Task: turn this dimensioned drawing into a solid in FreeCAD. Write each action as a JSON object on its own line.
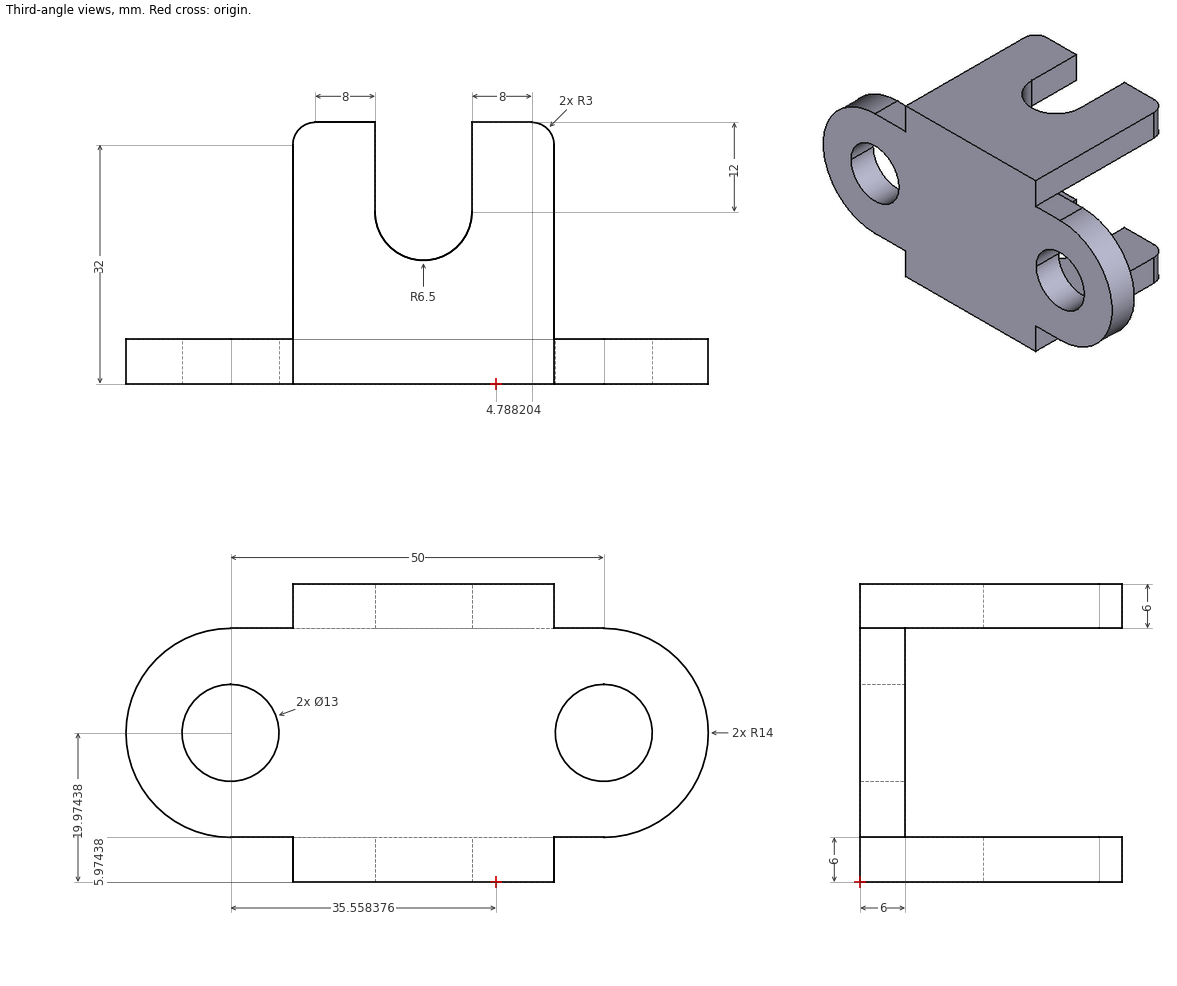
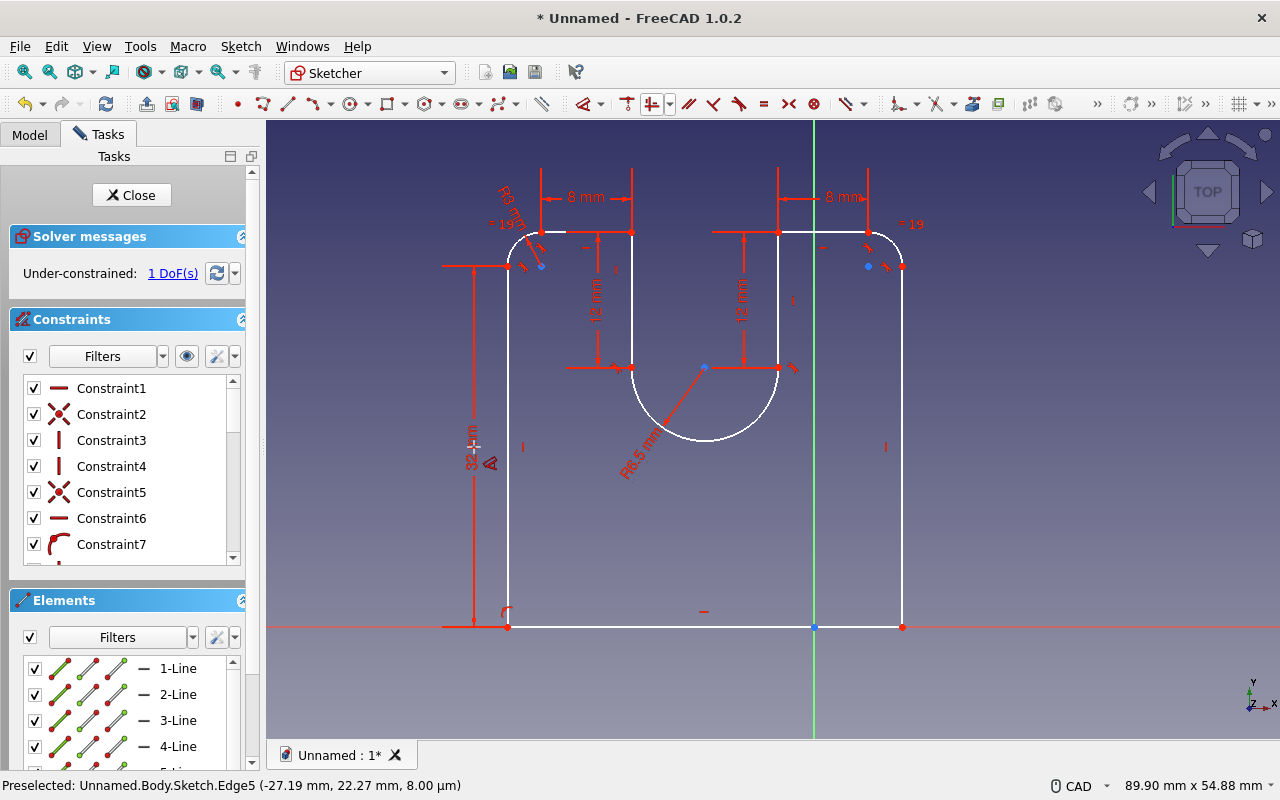
{"action": "left_click", "coordinate": [868, 232]}
{"action": "left_click", "coordinate": [841, 661]}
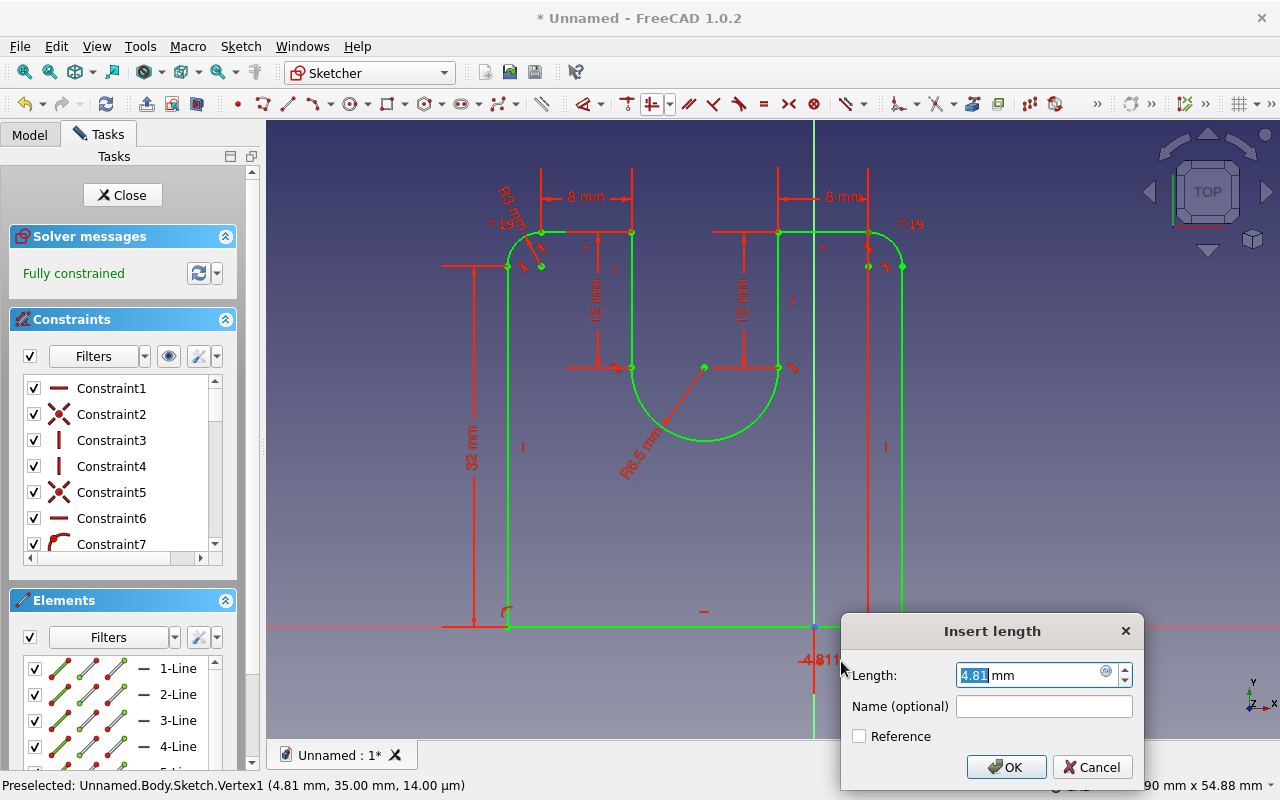
{"action": "type", "text": "4.788204"}
{"action": "key", "text": "Return"}
{"action": "key", "text": "Escape"}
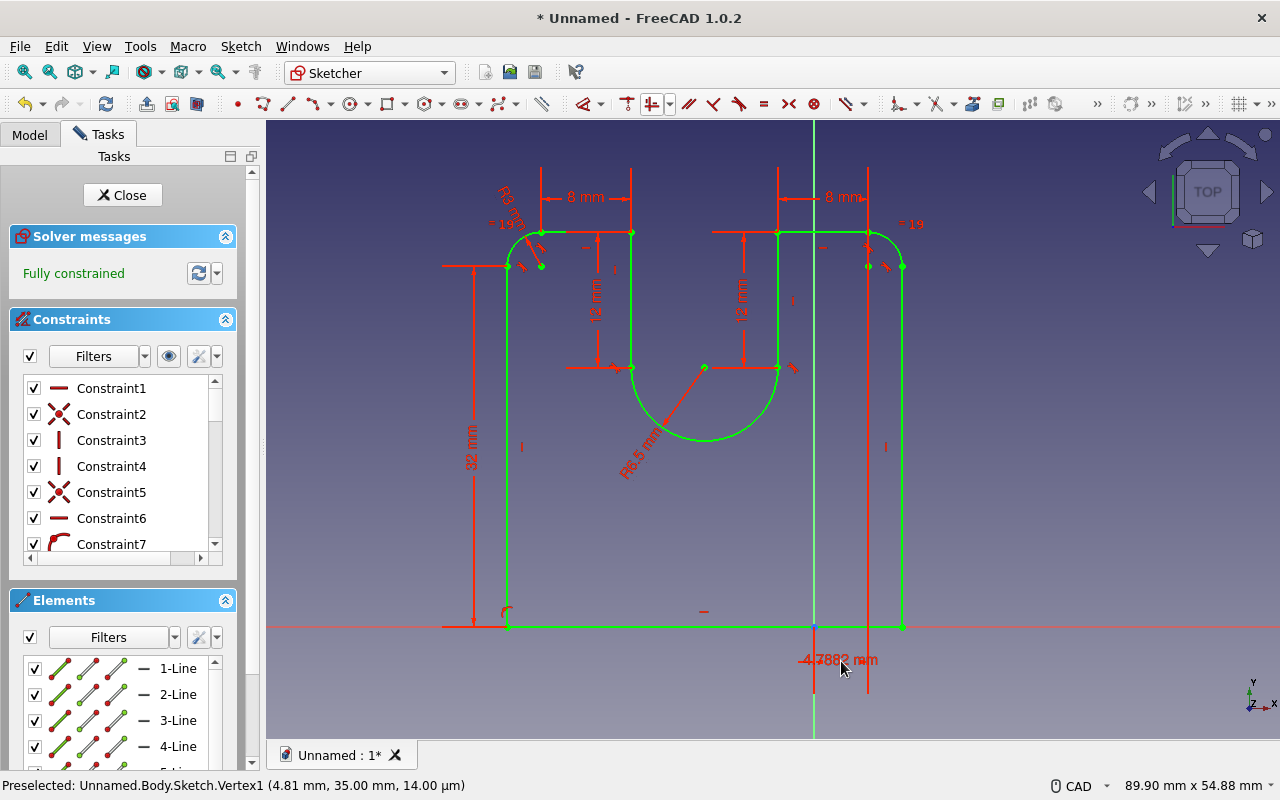
{"action": "left_click", "coordinate": [123, 195]}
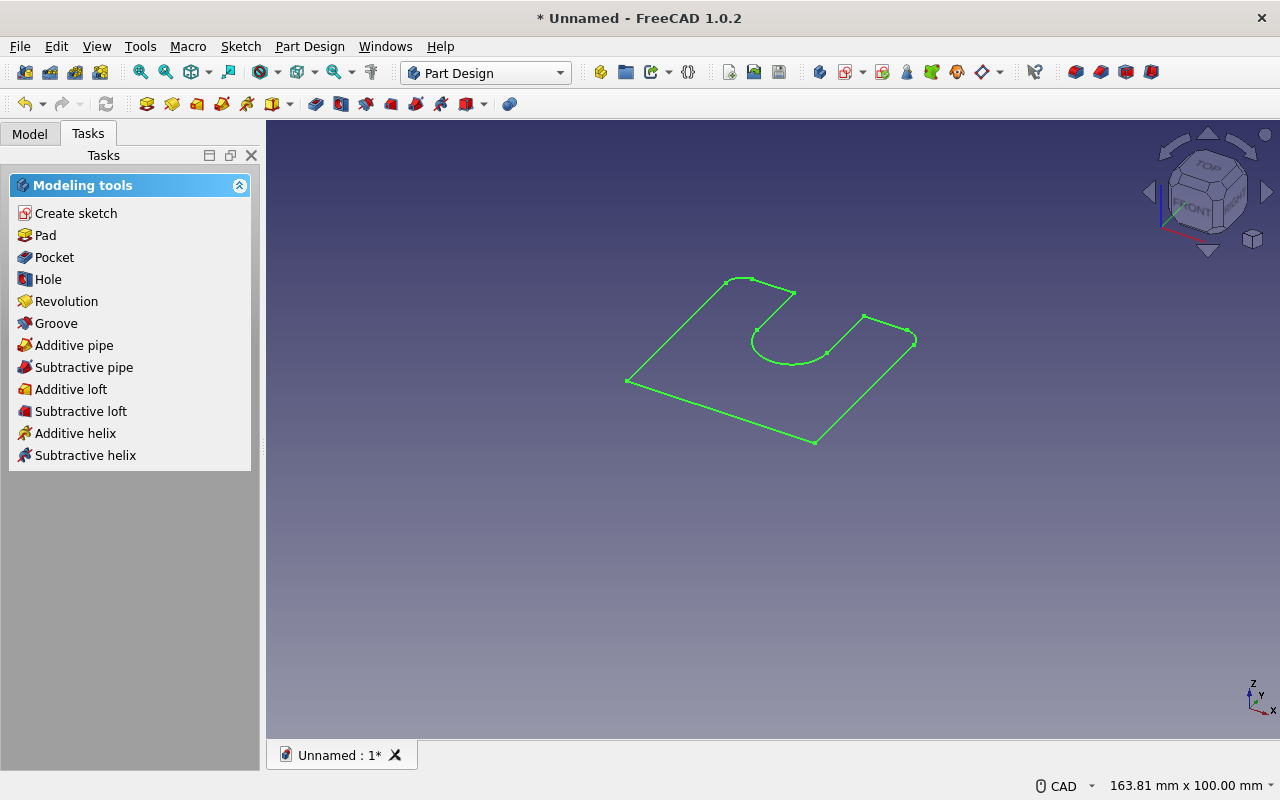
{"action": "left_click", "coordinate": [147, 104]}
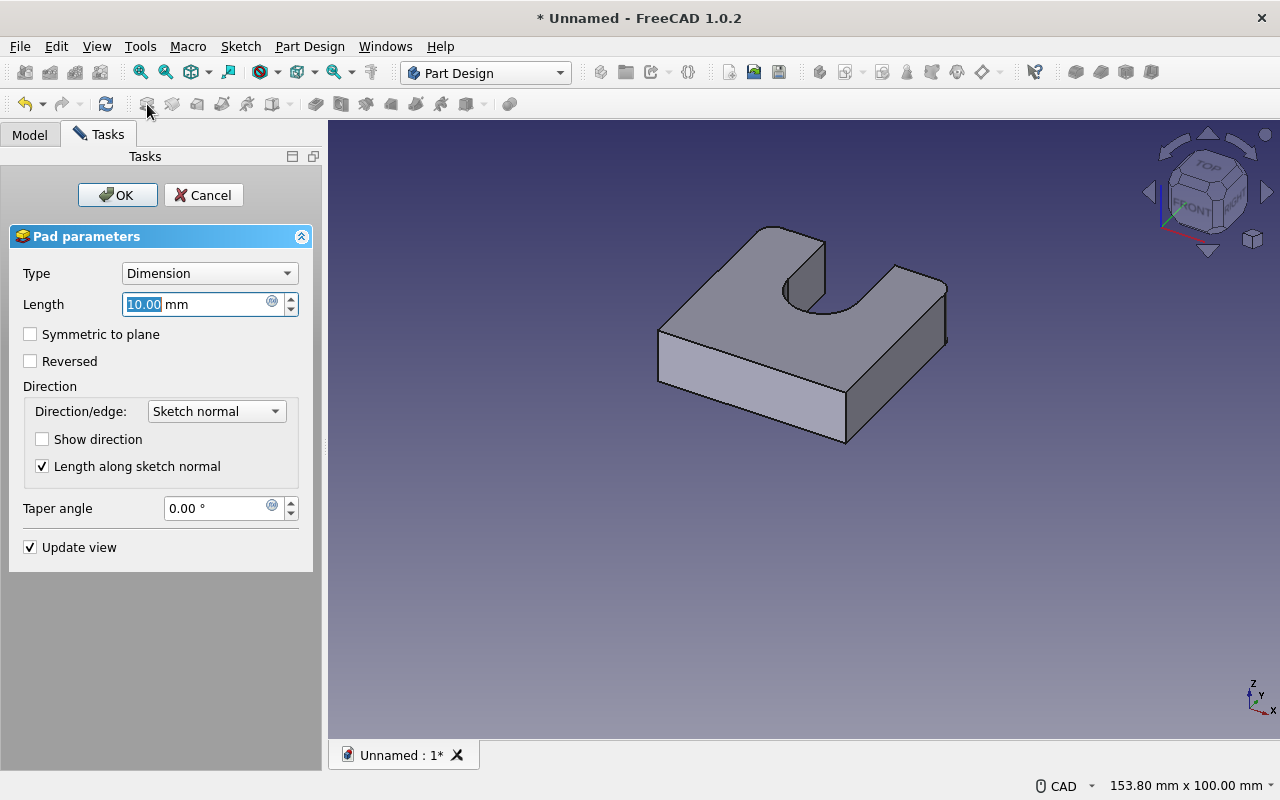
{"action": "type", "text": "6"}
{"action": "key", "text": "Tab"}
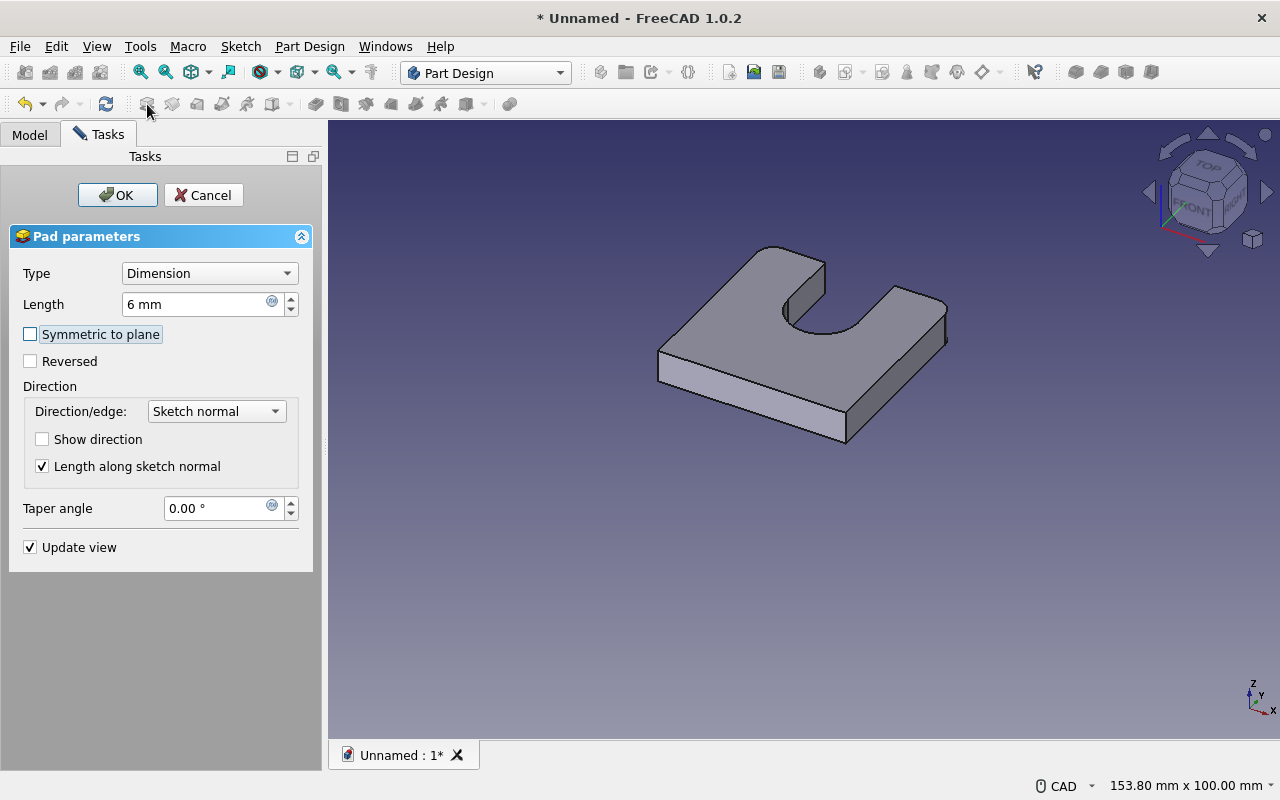
{"action": "left_click", "coordinate": [118, 195]}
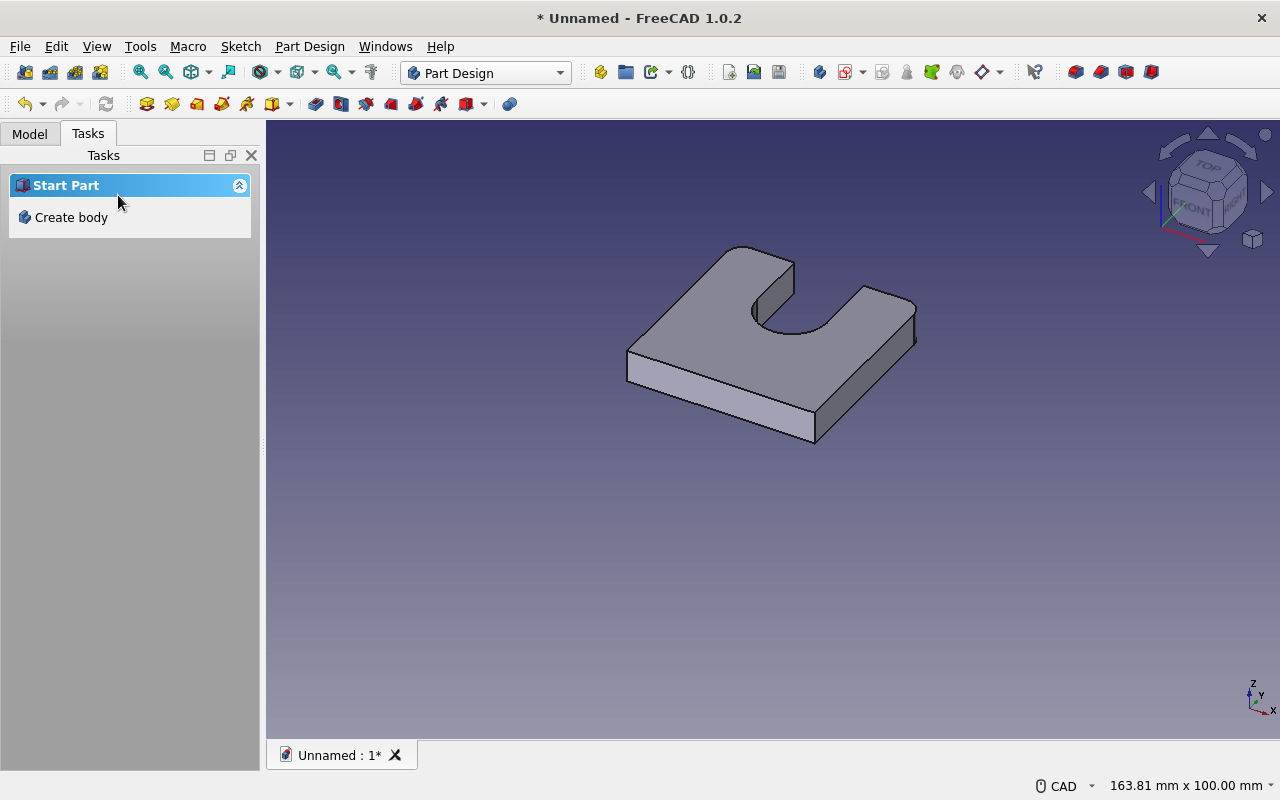
{"action": "left_click", "coordinate": [141, 72]}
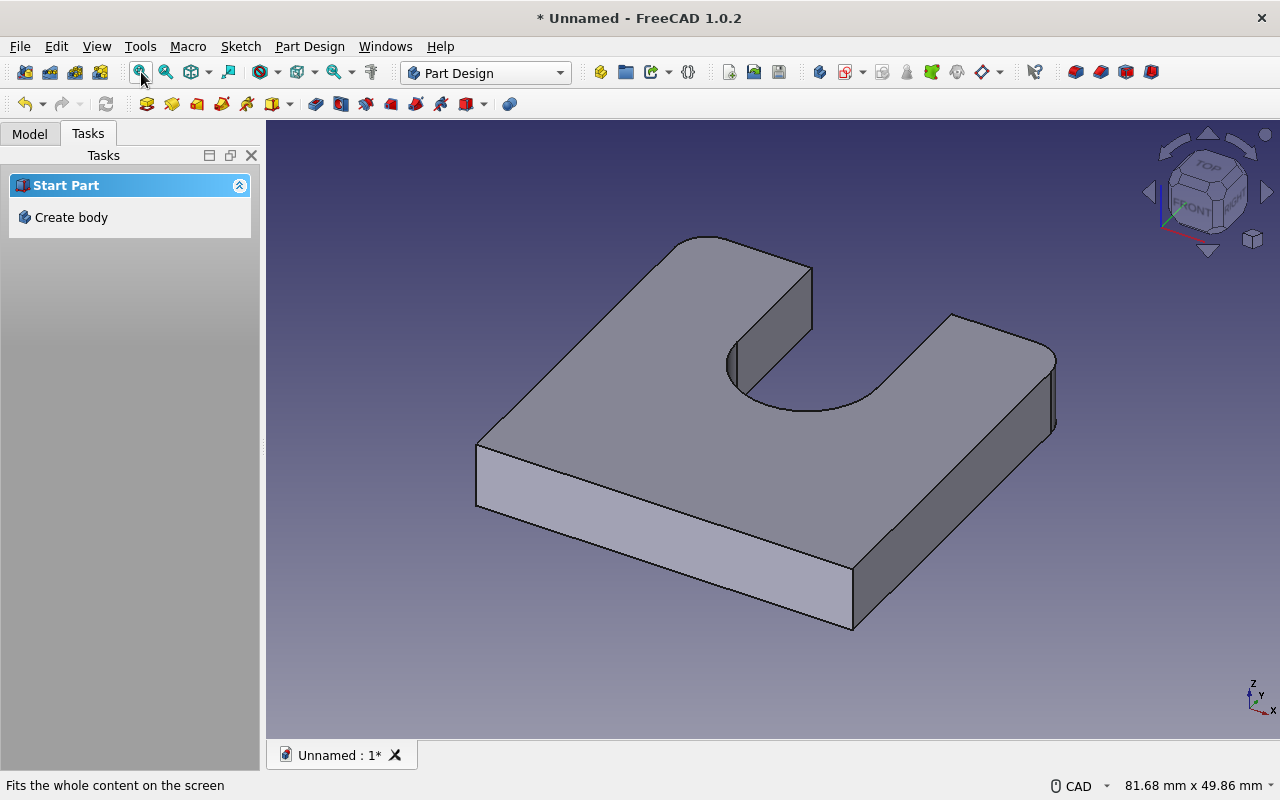
{"action": "left_click", "coordinate": [772, 572]}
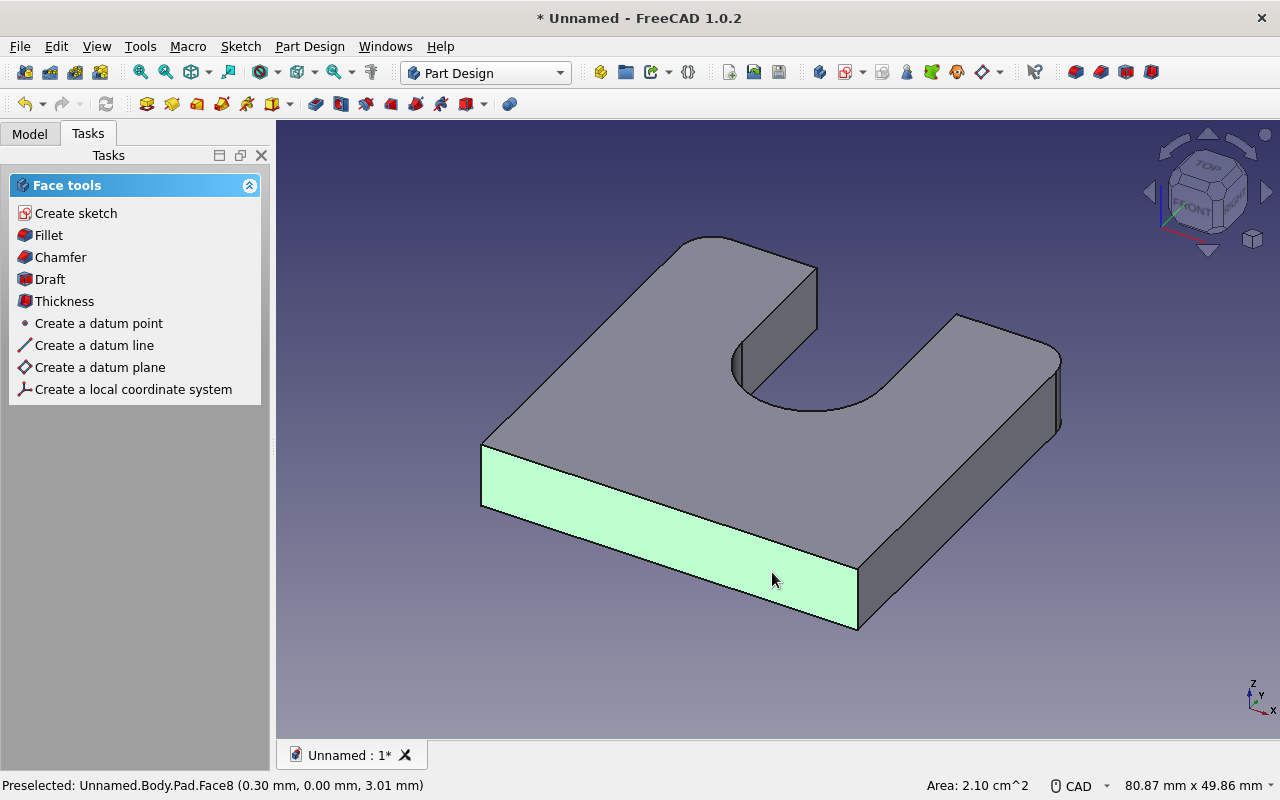
{"action": "left_click", "coordinate": [844, 72]}